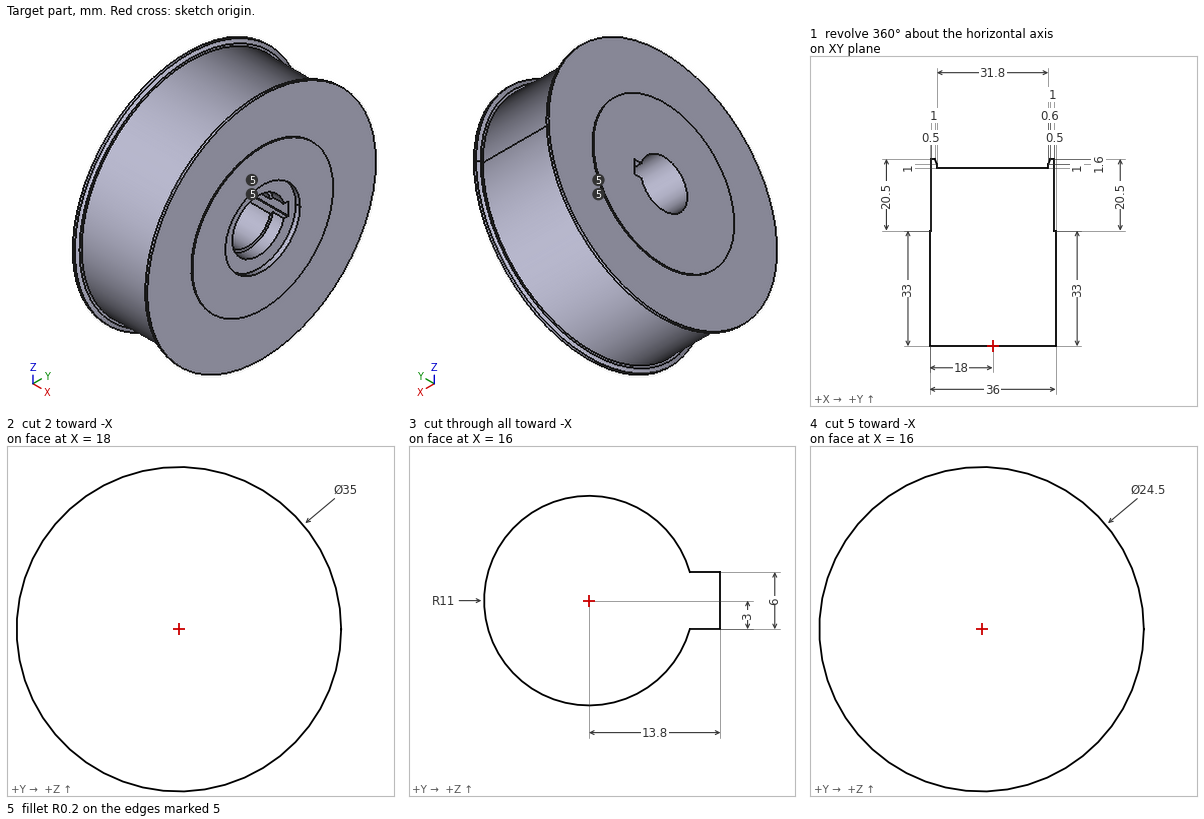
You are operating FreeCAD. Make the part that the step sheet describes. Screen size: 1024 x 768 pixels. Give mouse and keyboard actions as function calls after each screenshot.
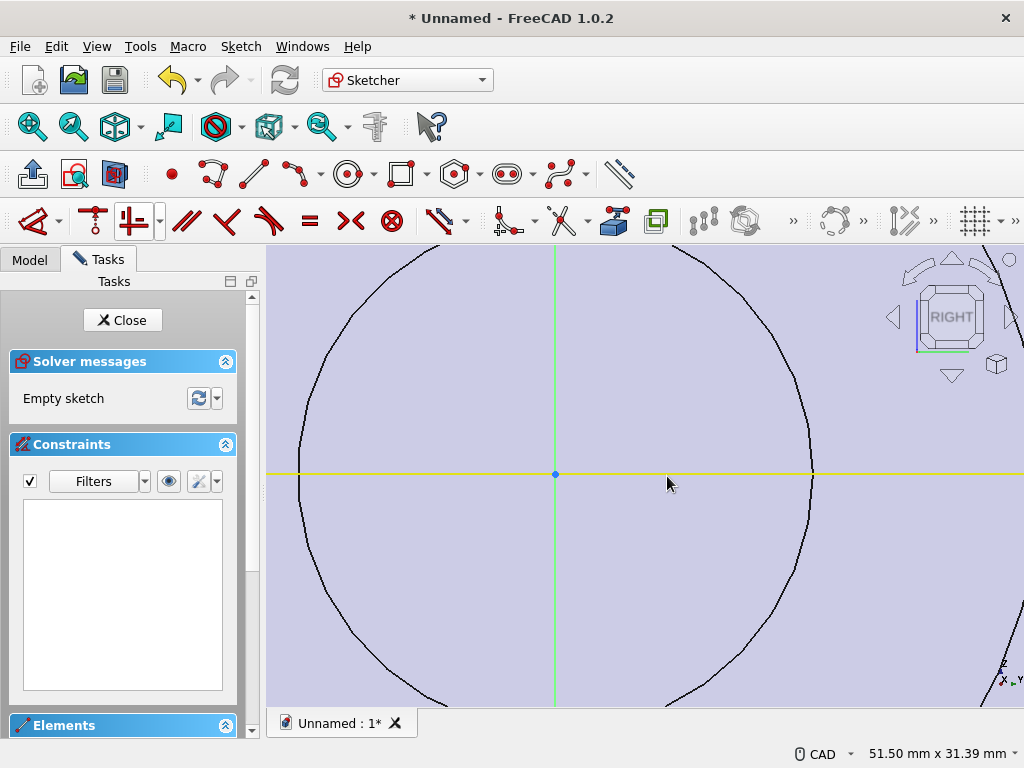
key(g)
key(m)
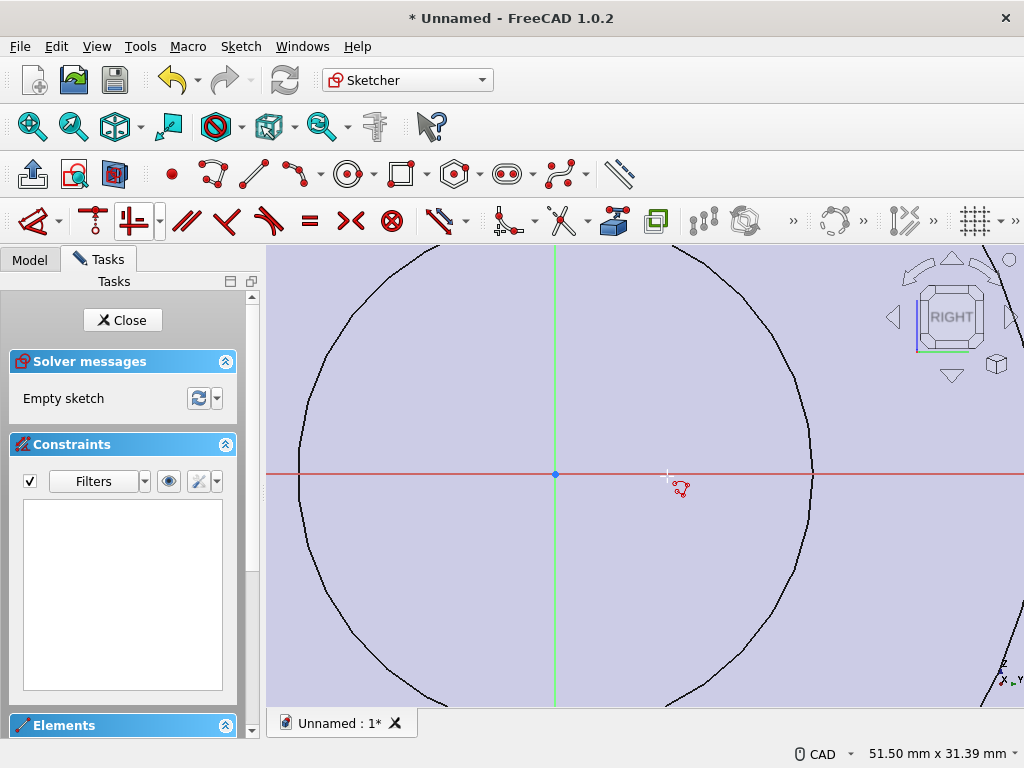
click(711, 518)
click(758, 518)
click(758, 430)
click(711, 430)
right_click(711, 430)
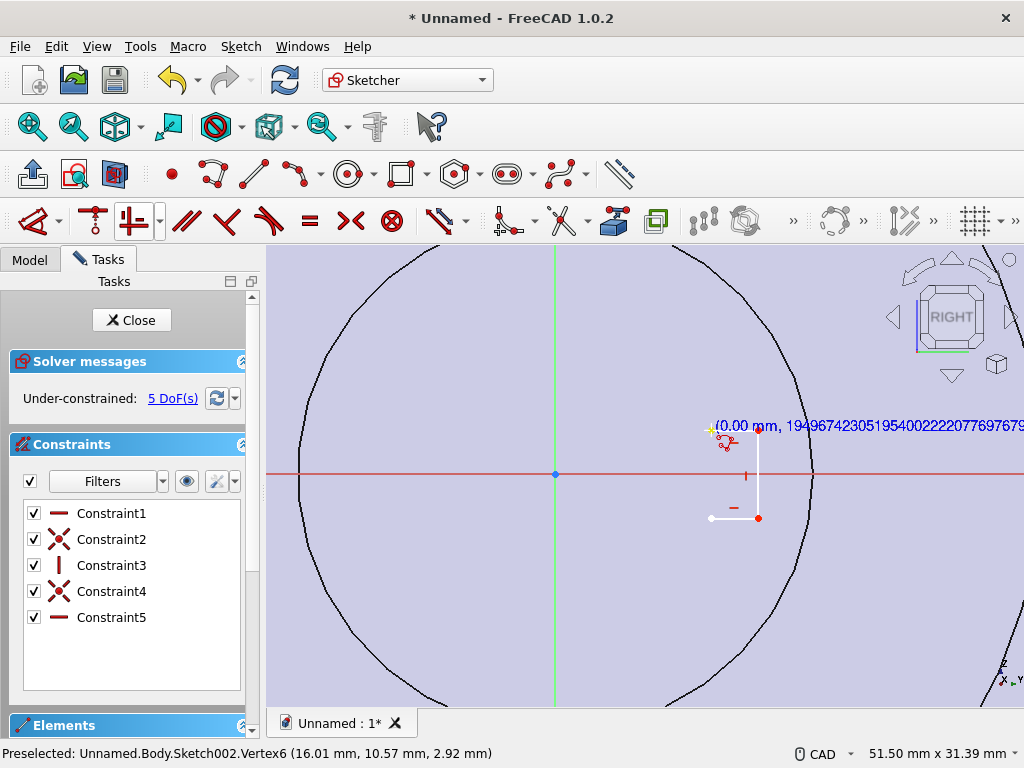
key(g)
key(3)
key(a)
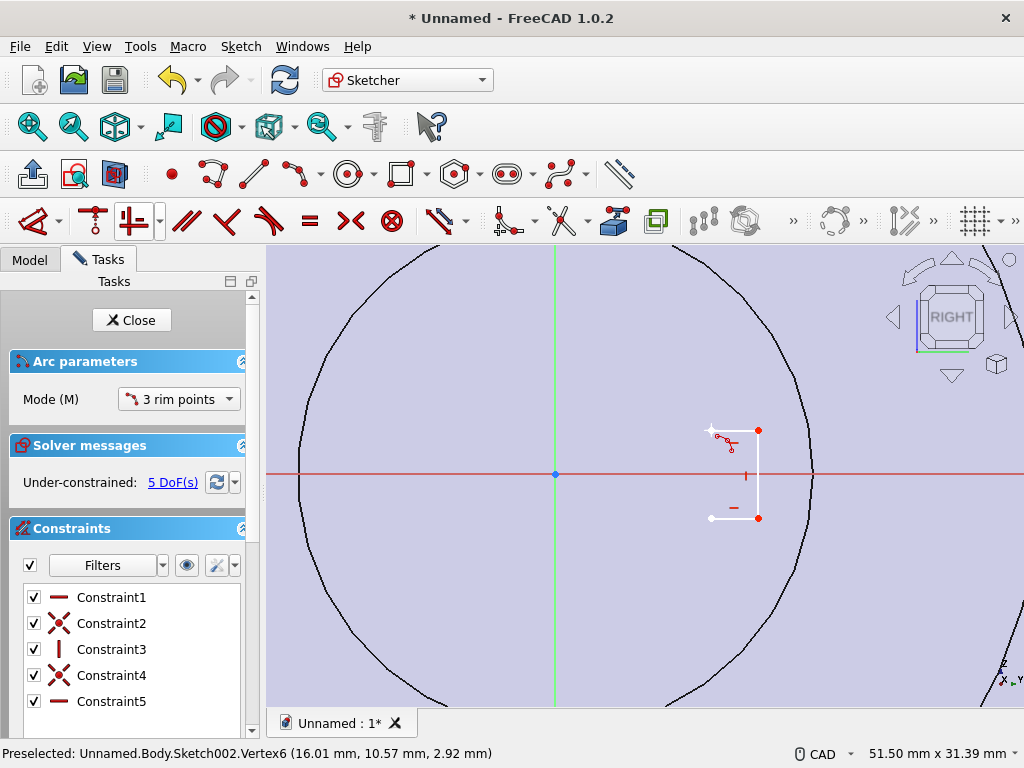
click(711, 431)
click(711, 519)
click(419, 386)
key(Escape)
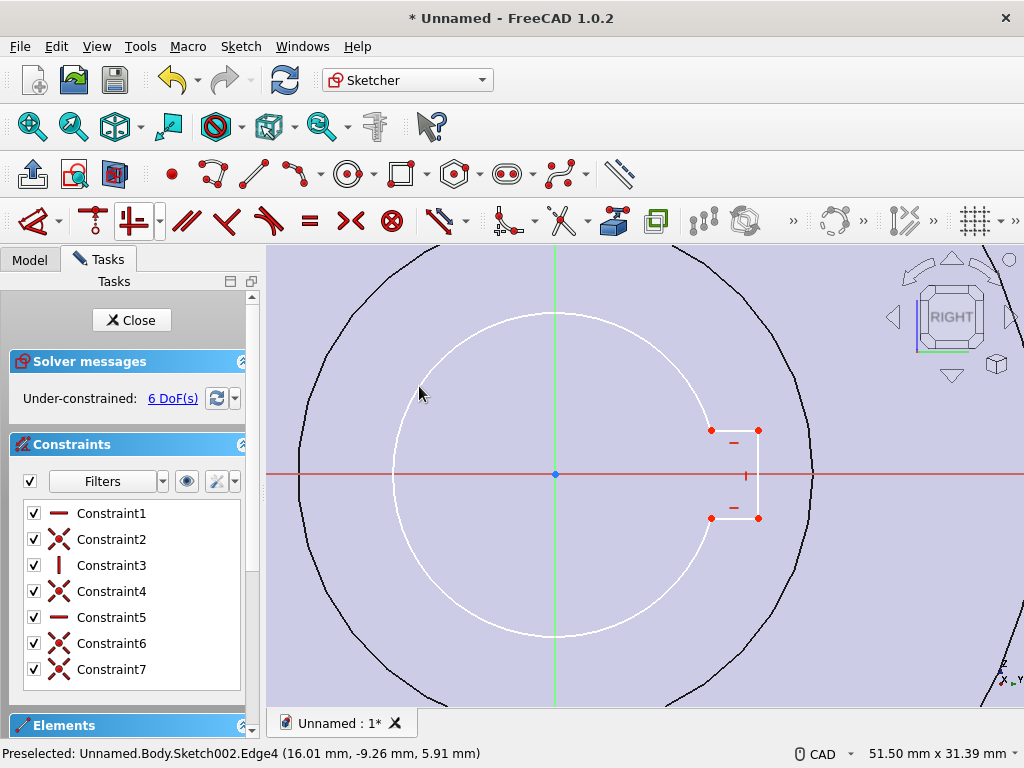
drag(545, 464, 565, 485)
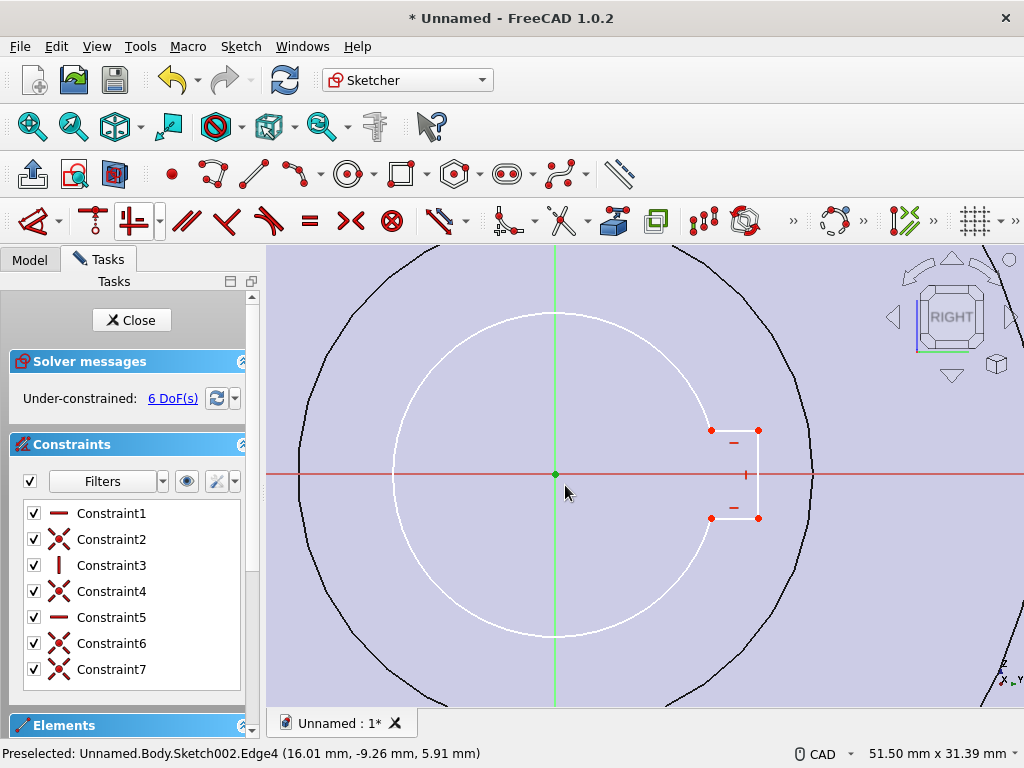
key(c)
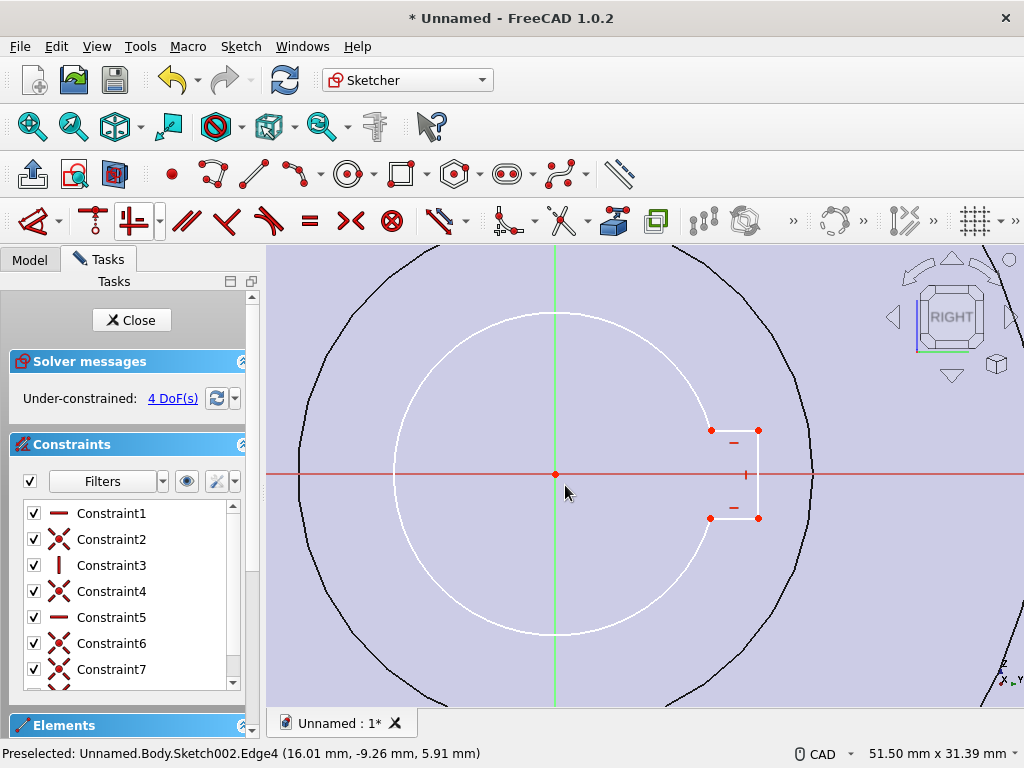
key(d)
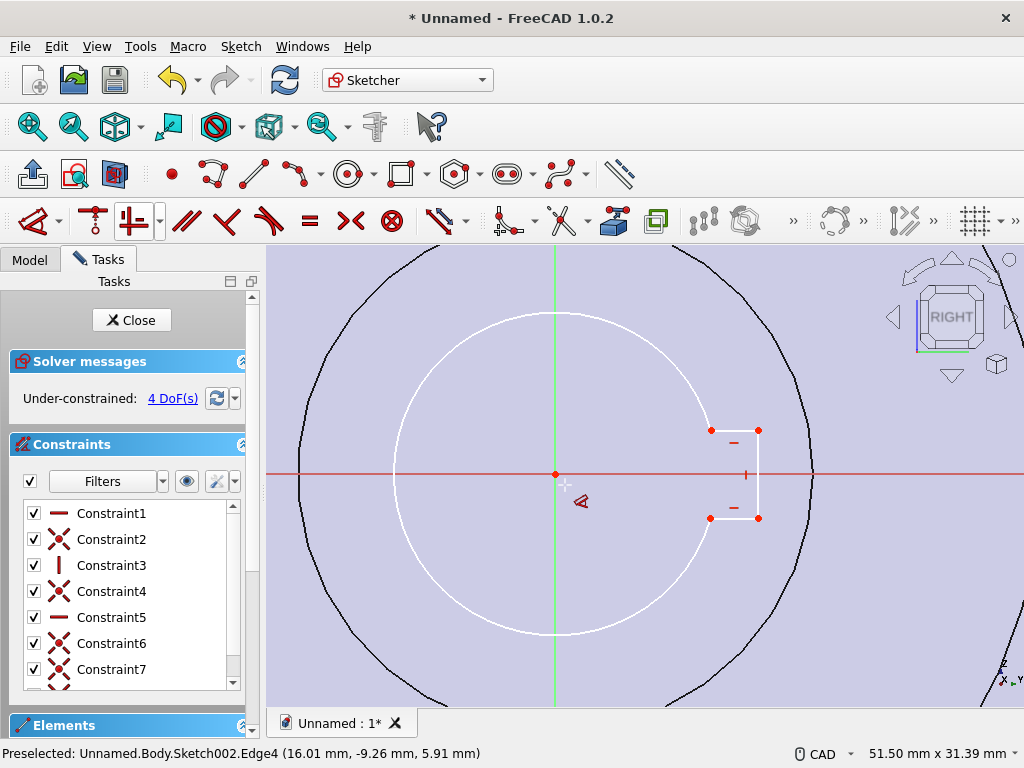
click(490, 326)
click(477, 297)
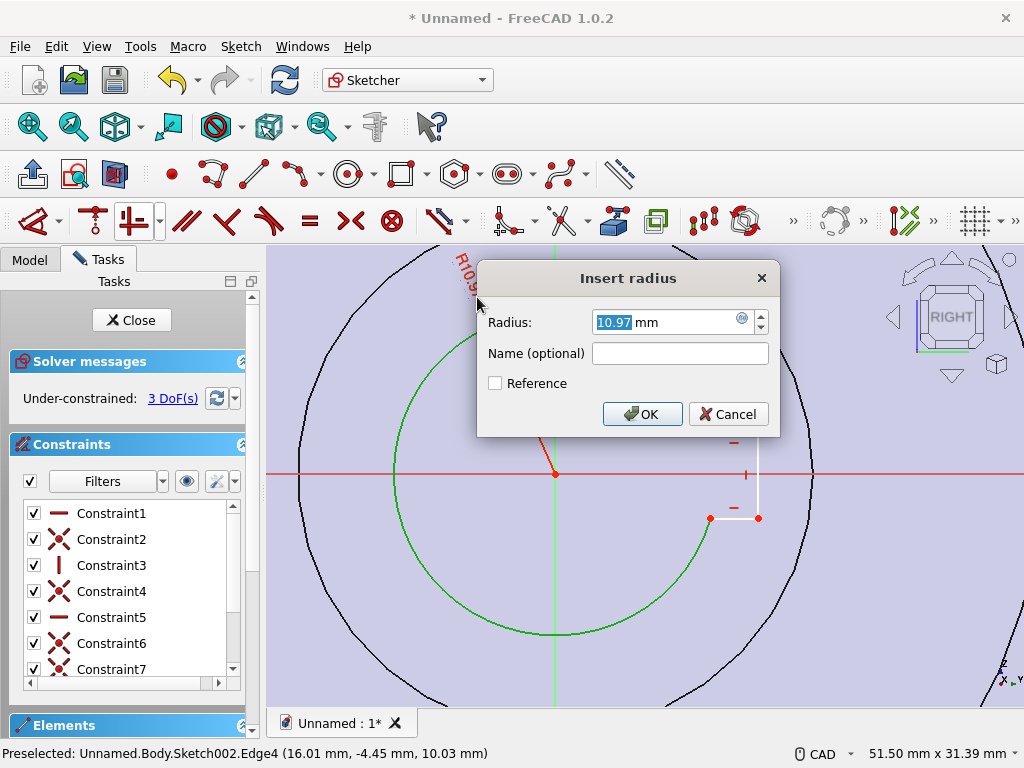
text(11)
key(Return)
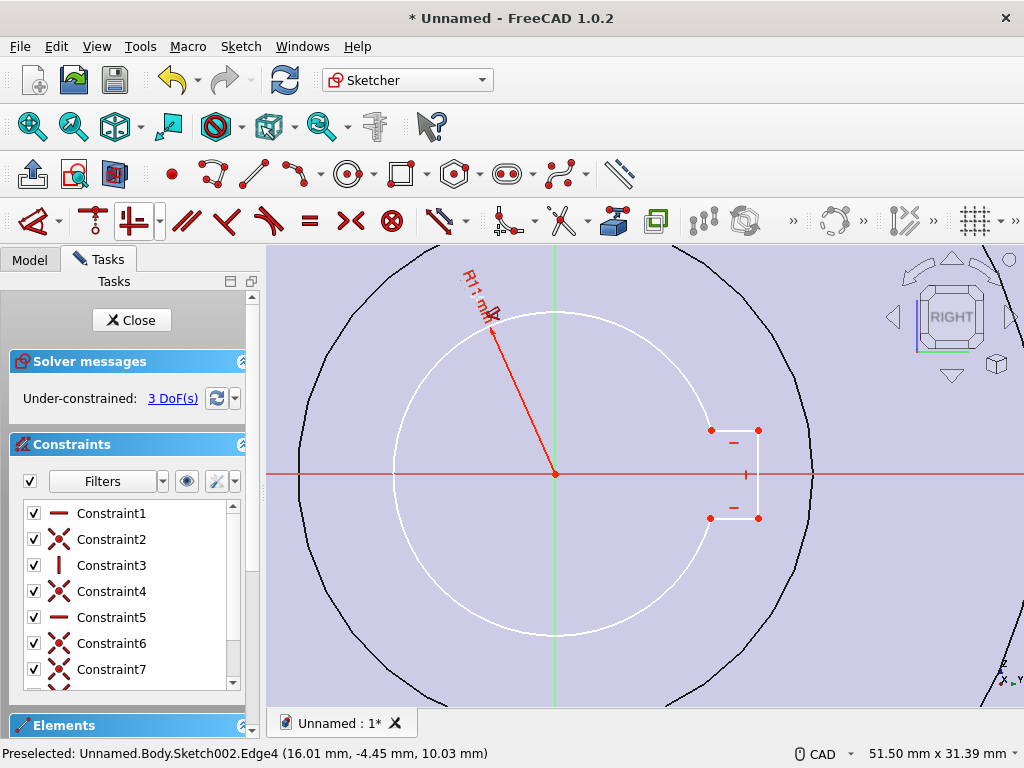
click(758, 493)
click(792, 455)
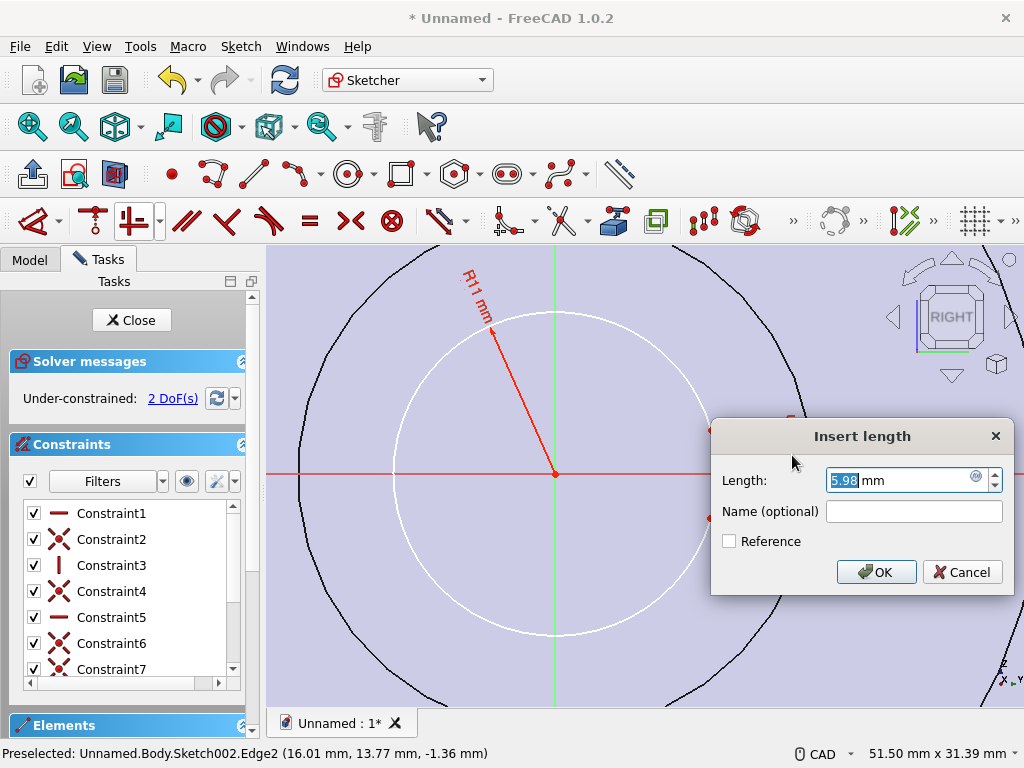
text(6)
key(Return)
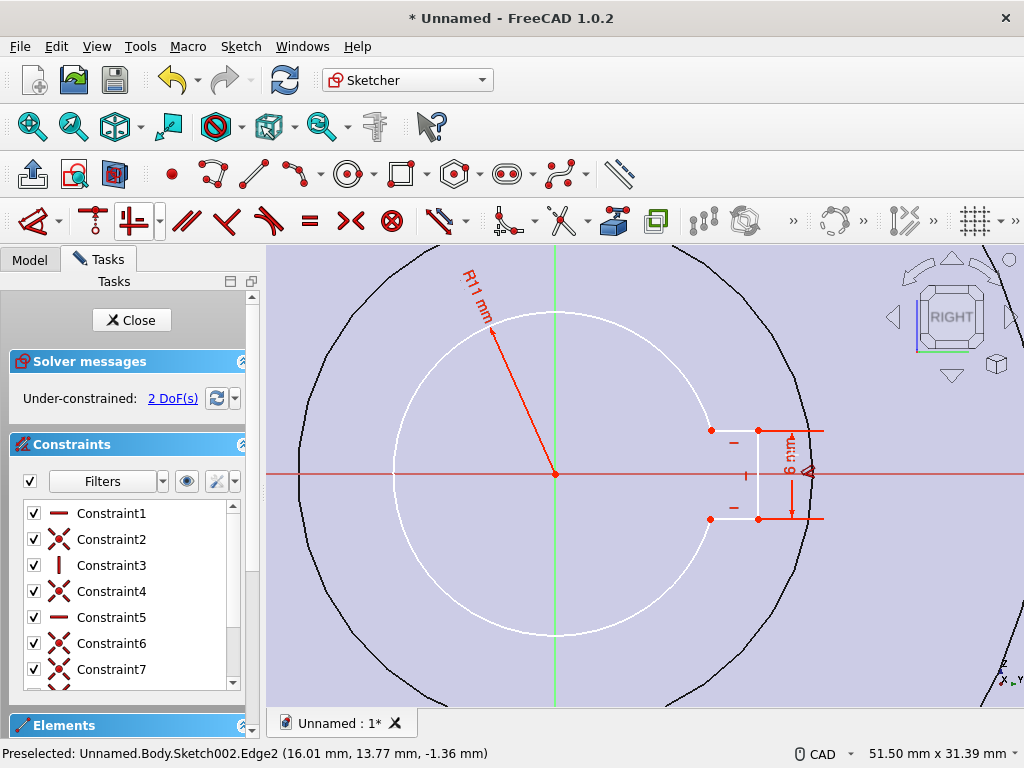
click(711, 519)
click(745, 497)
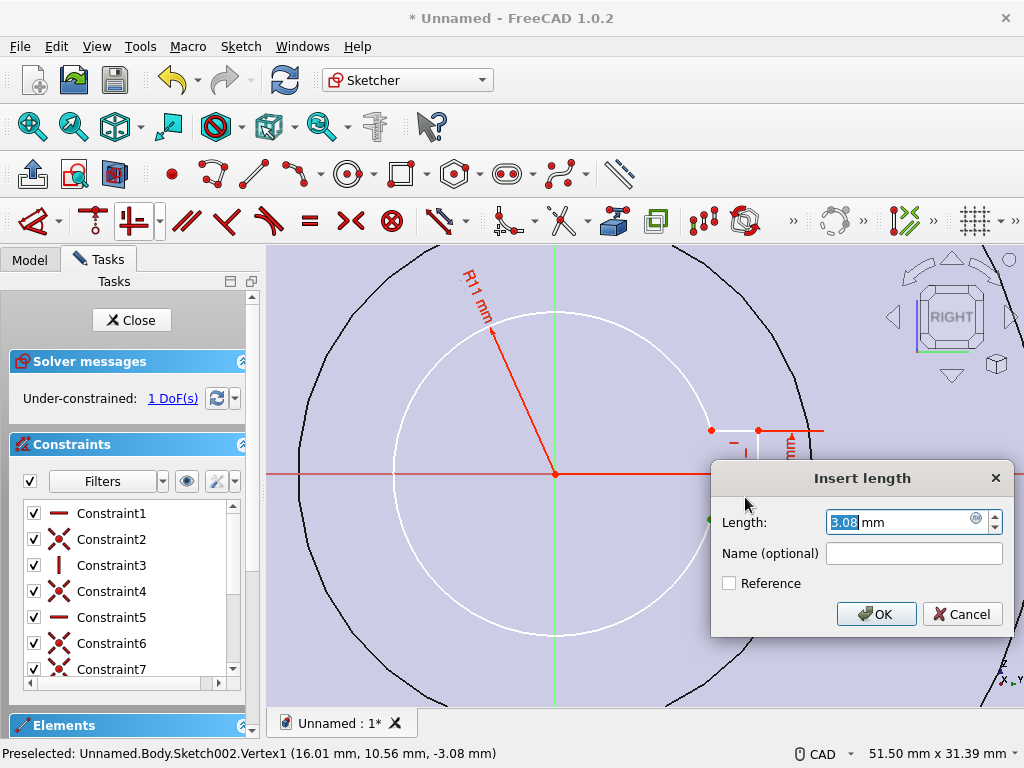
text(3)
key(Return)